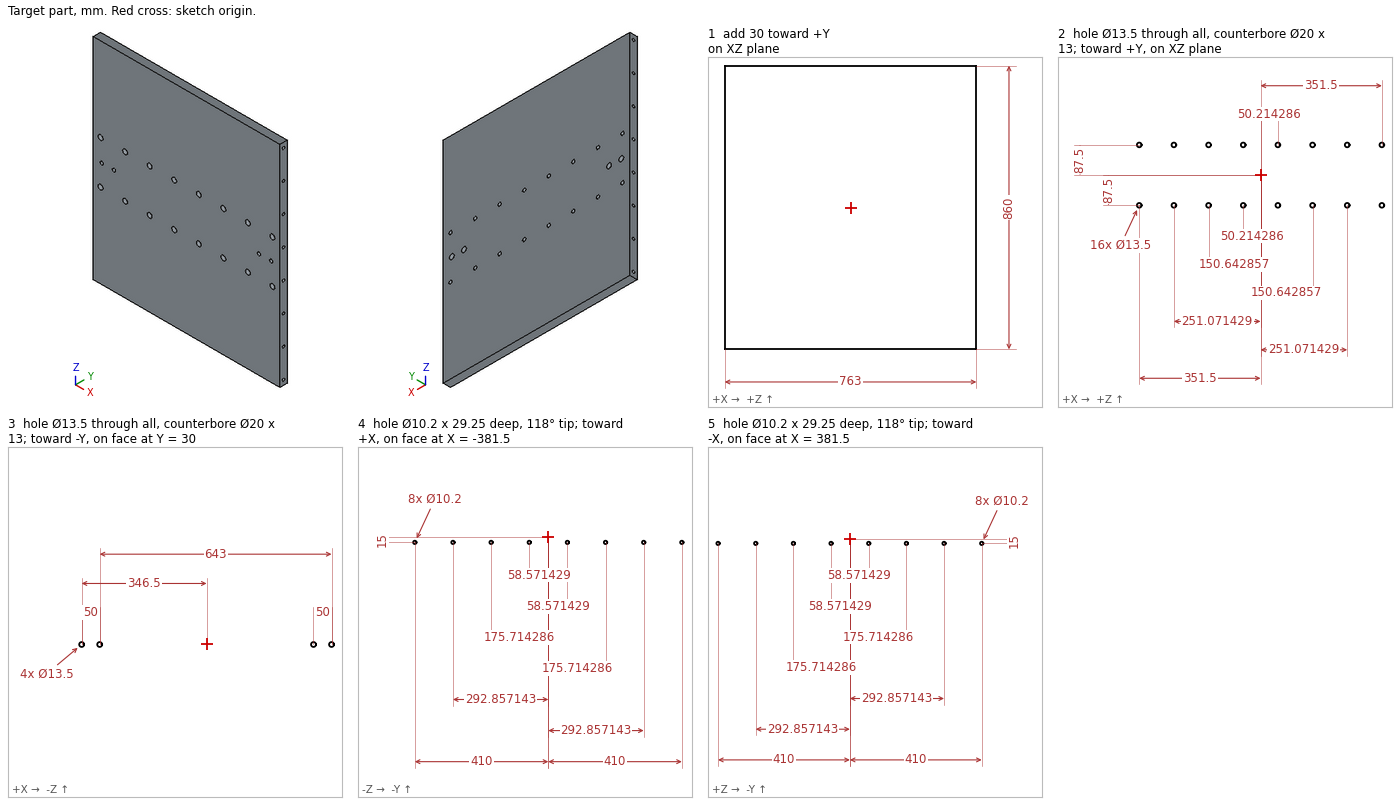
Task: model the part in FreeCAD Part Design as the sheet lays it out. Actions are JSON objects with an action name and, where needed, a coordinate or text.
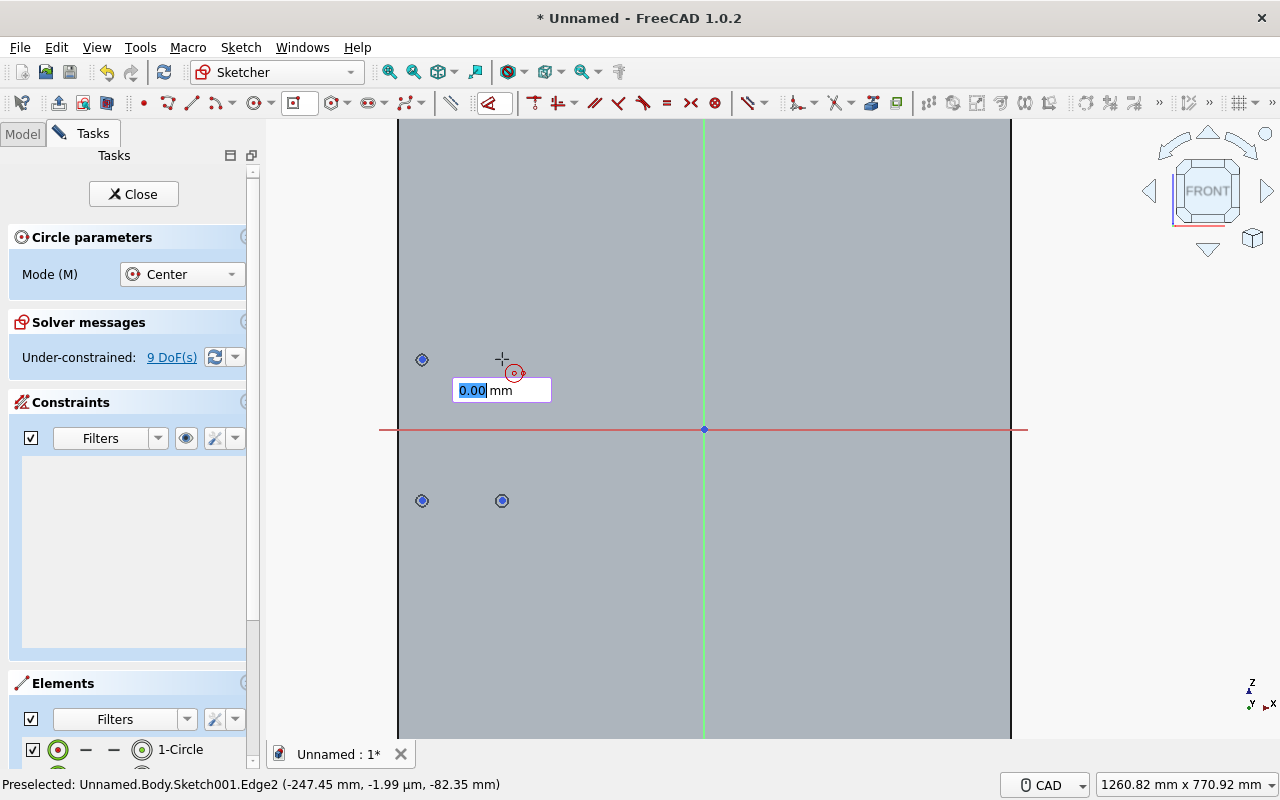
{"action": "scroll", "coordinate": [506, 355], "scroll_direction": "up", "scroll_amount": 6}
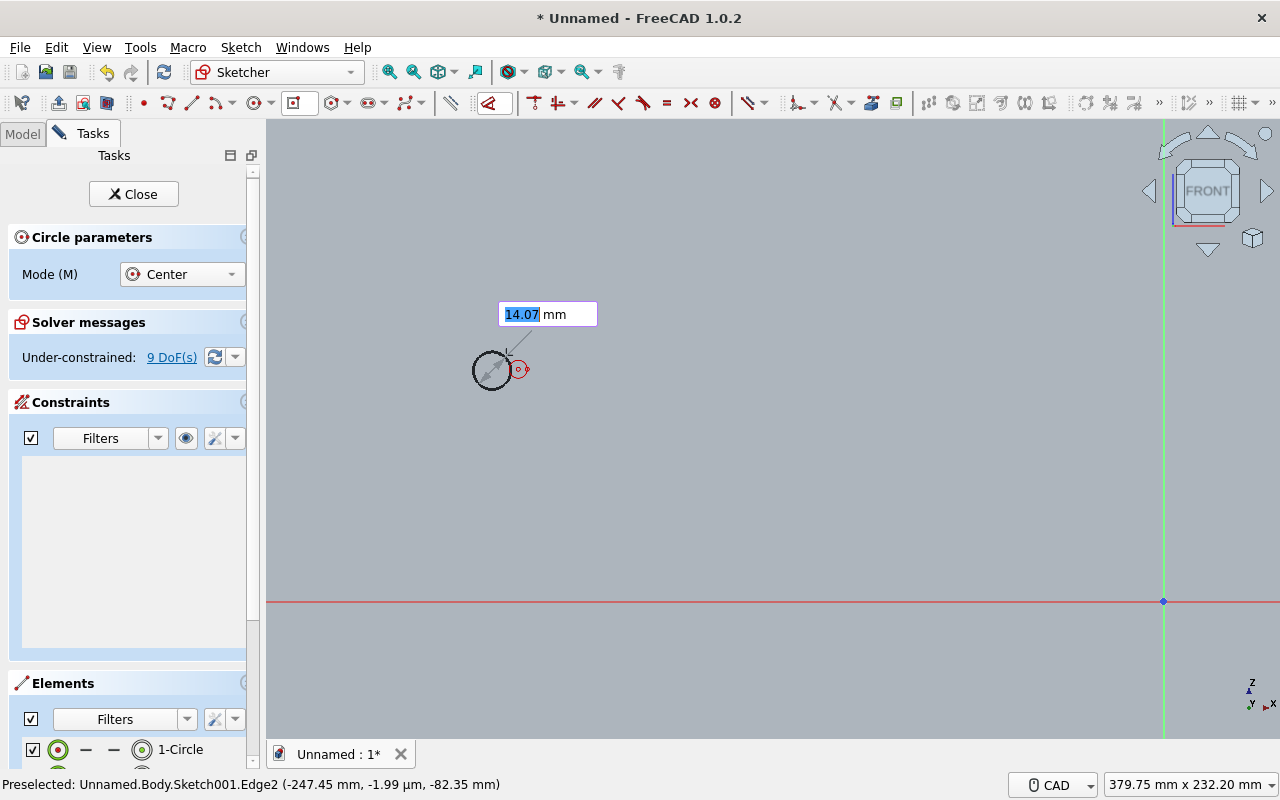
{"action": "left_click", "coordinate": [506, 355]}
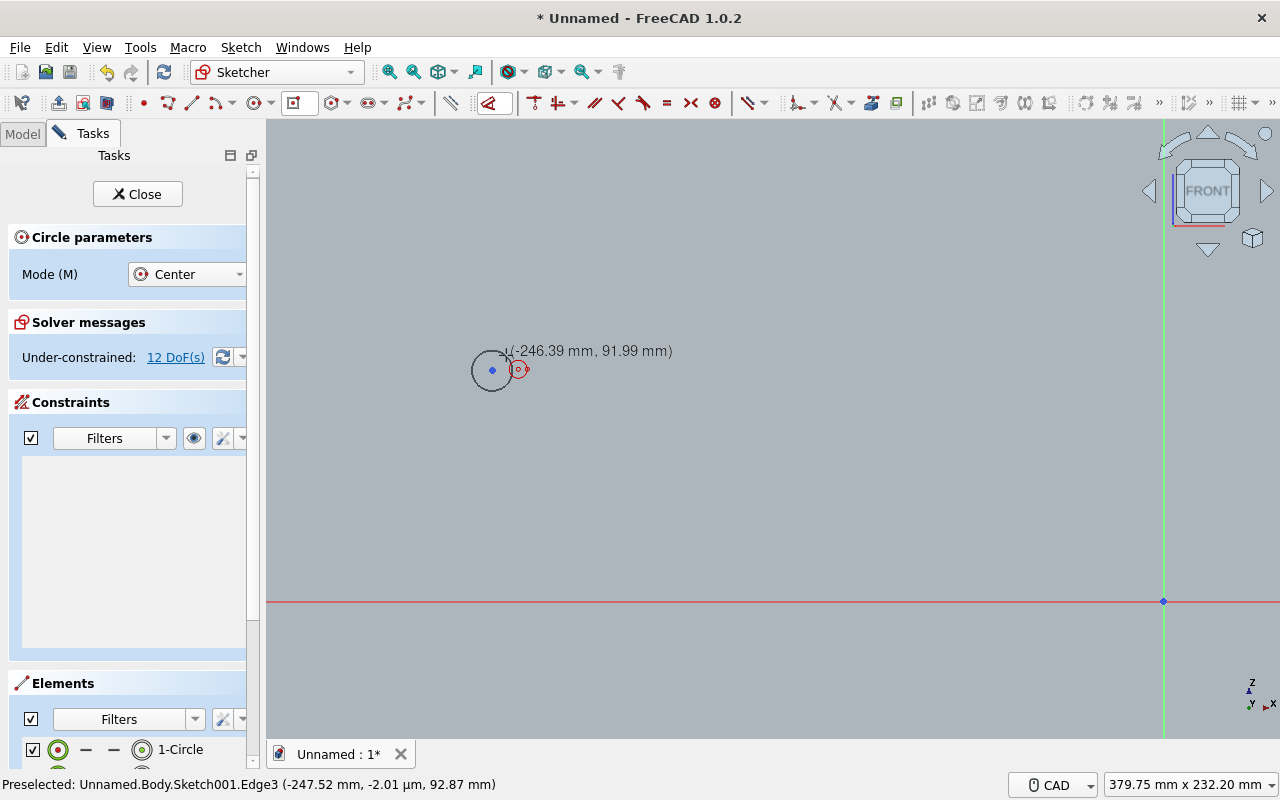
{"action": "scroll", "coordinate": [506, 355], "scroll_direction": "down", "scroll_amount": 6}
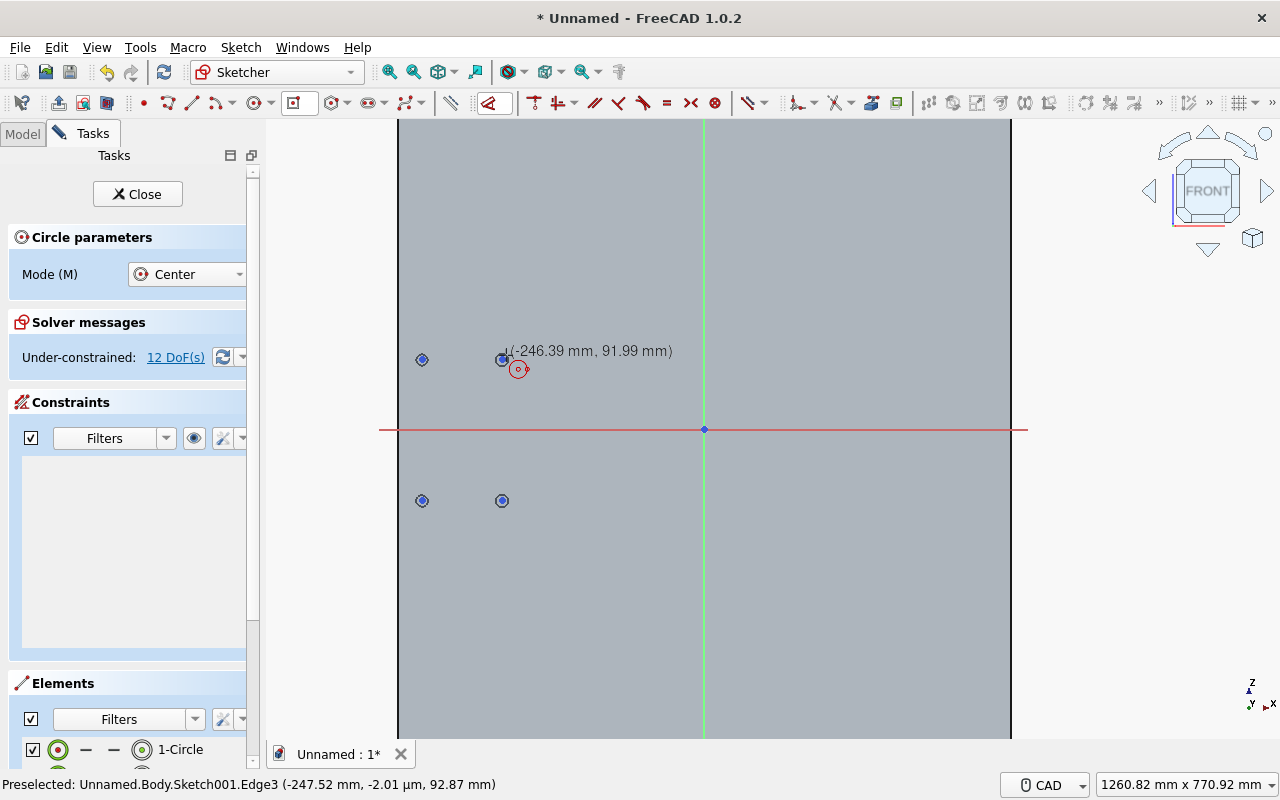
{"action": "scroll", "coordinate": [583, 500], "scroll_direction": "up", "scroll_amount": 8}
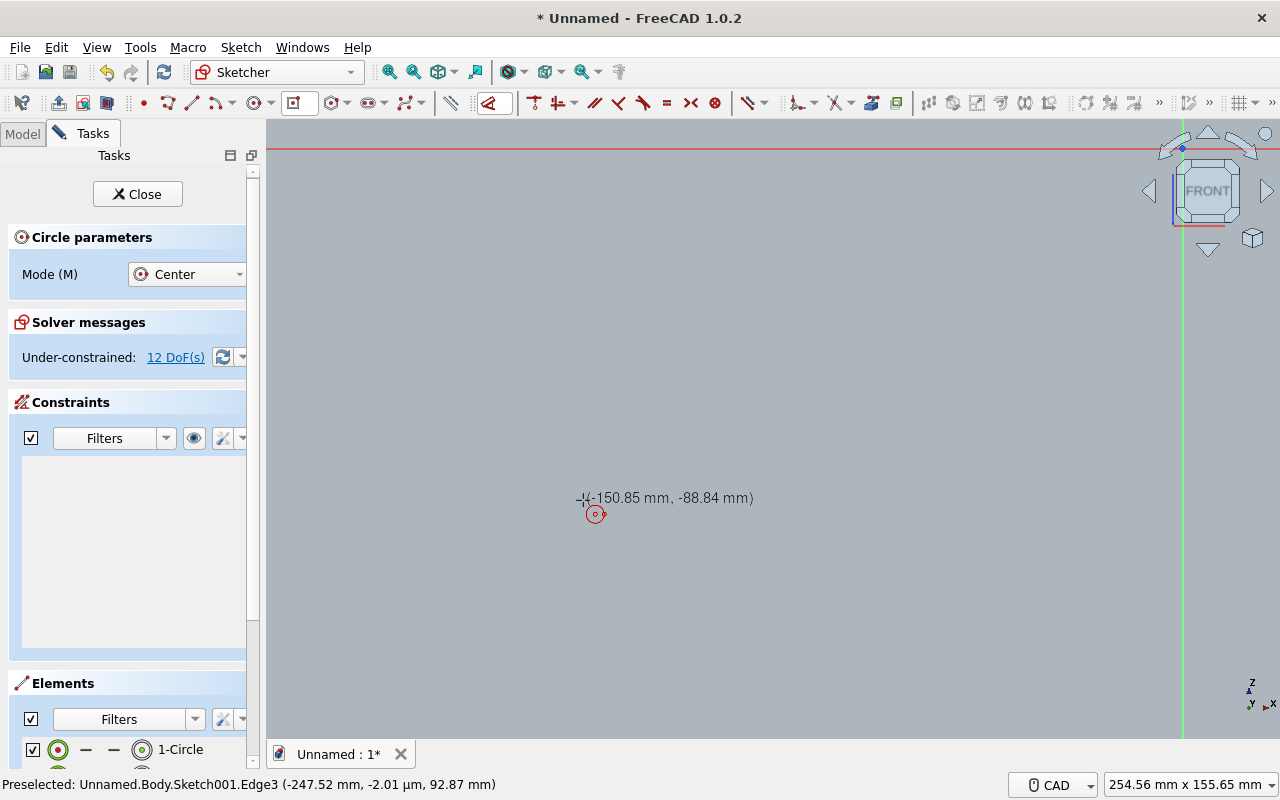
{"action": "scroll", "coordinate": [584, 500], "scroll_direction": "down", "scroll_amount": 8}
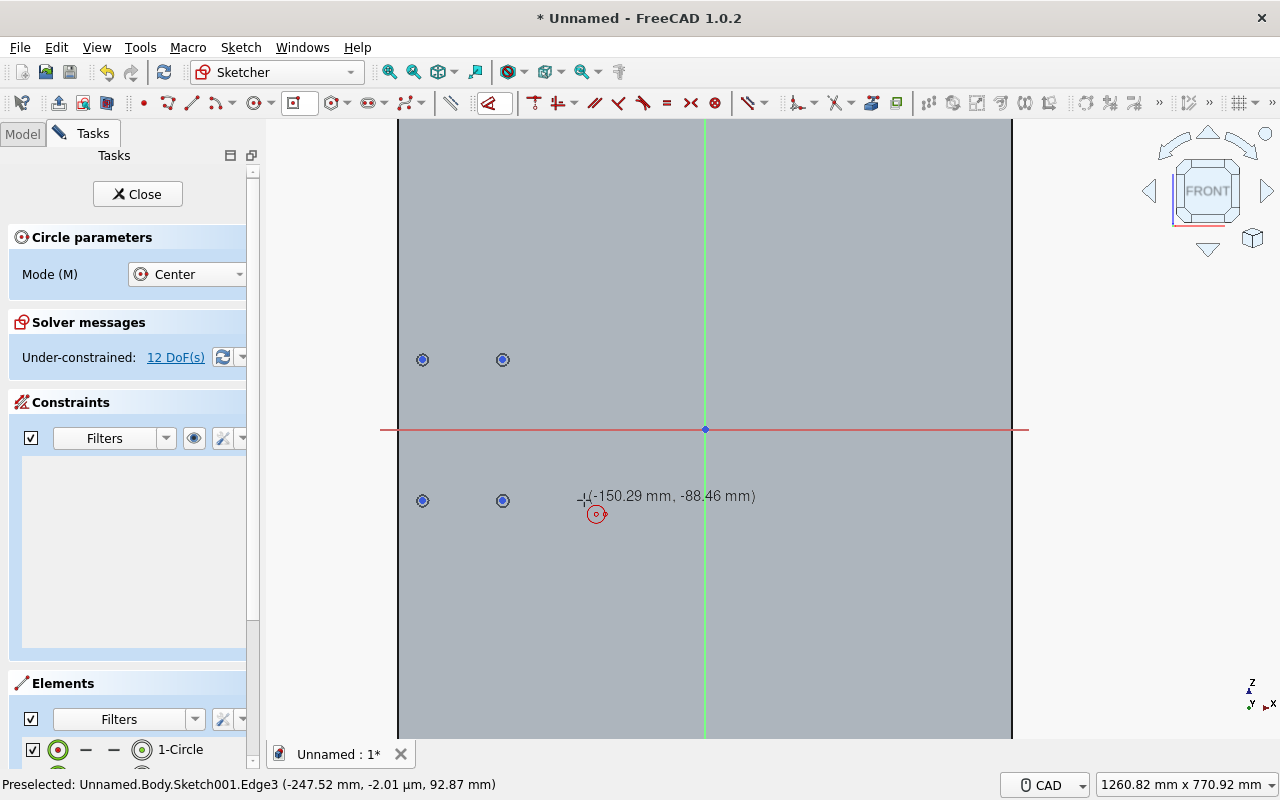
{"action": "left_click", "coordinate": [584, 500]}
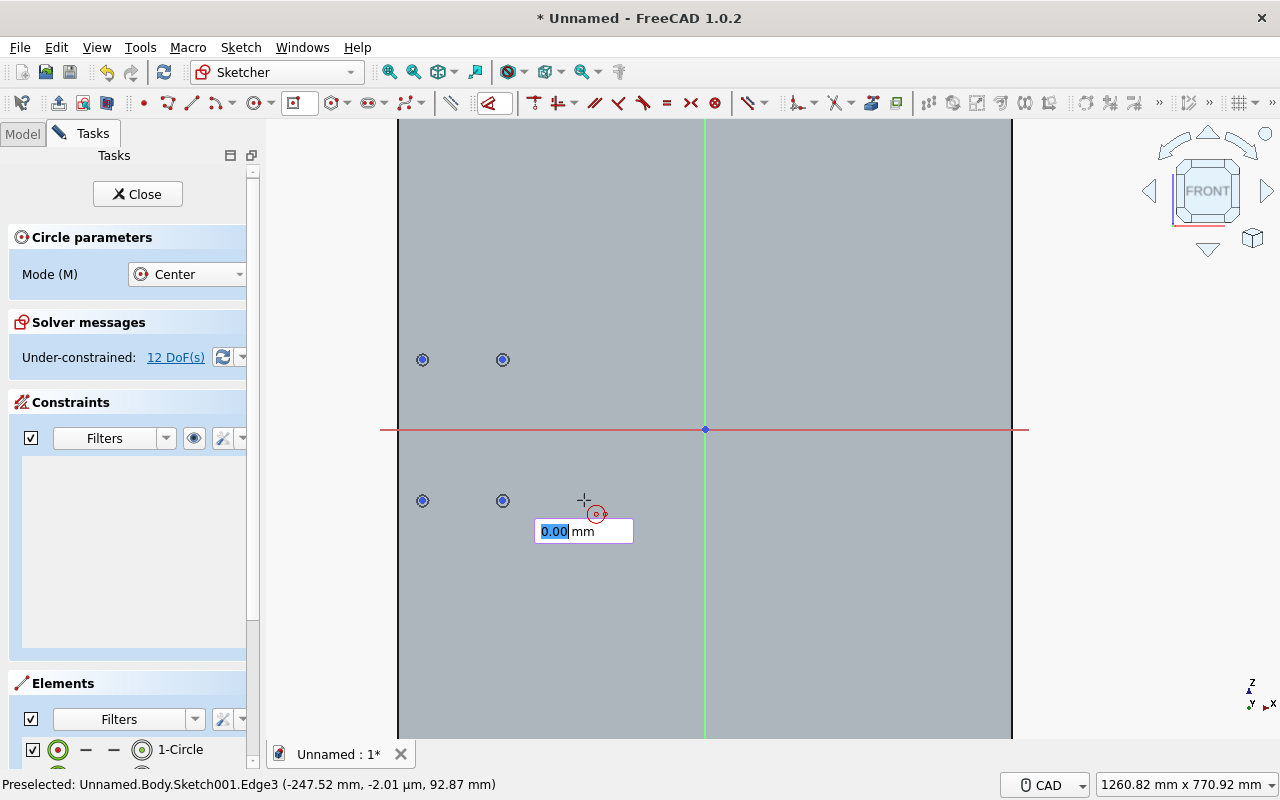
{"action": "scroll", "coordinate": [588, 496], "scroll_direction": "up", "scroll_amount": 6}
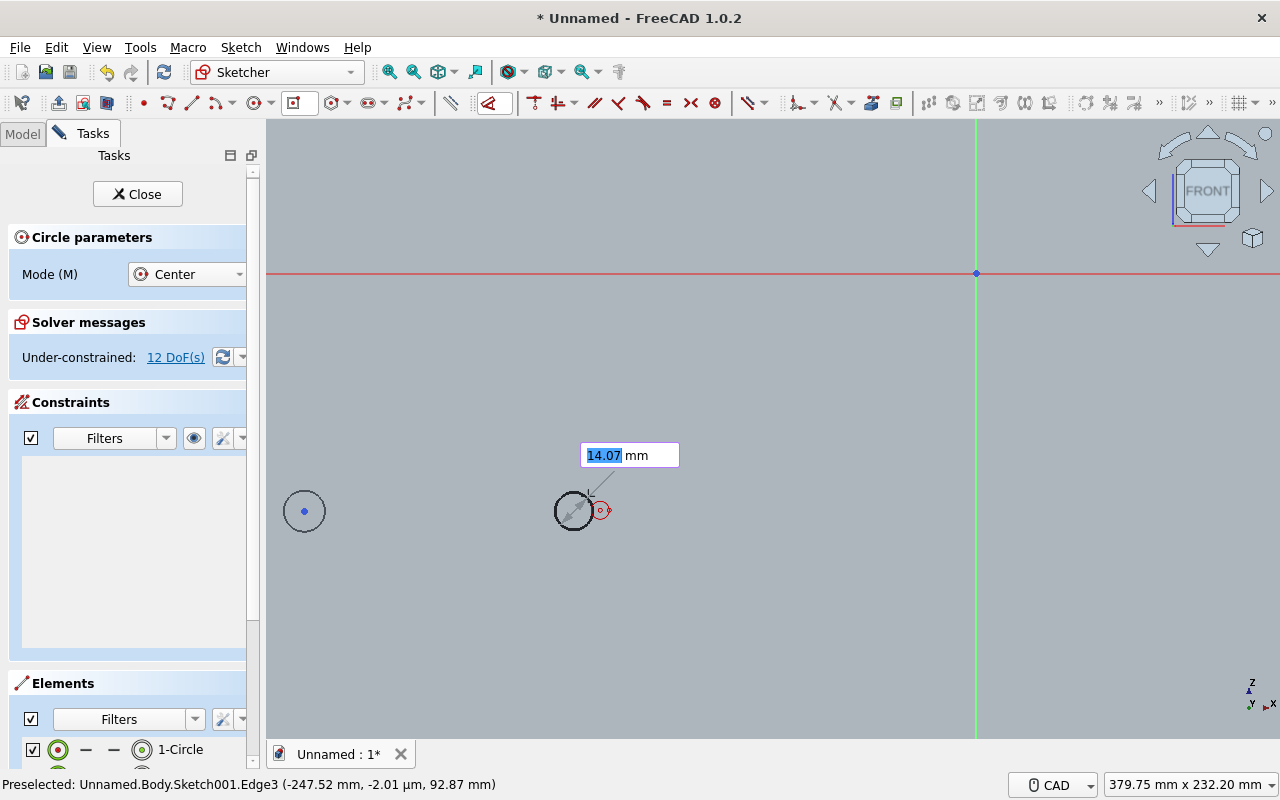
{"action": "left_click", "coordinate": [587, 495]}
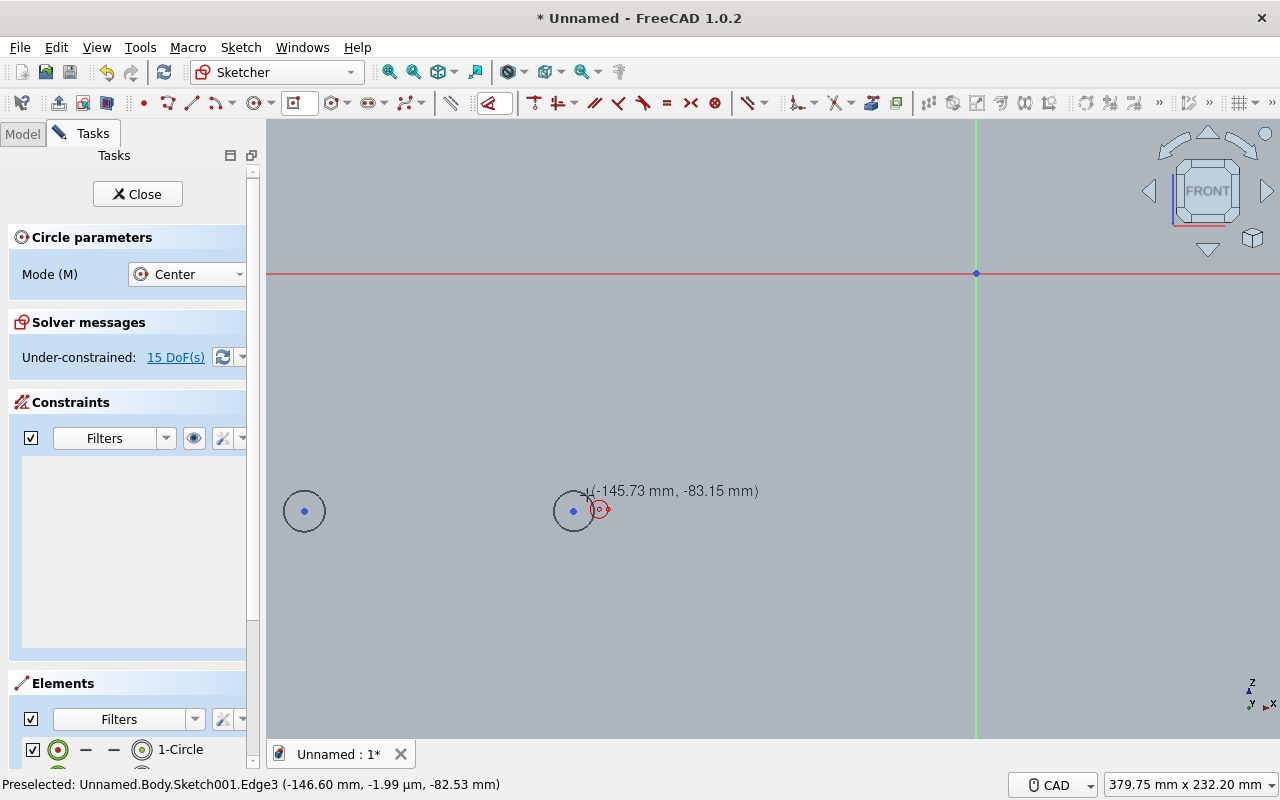
{"action": "scroll", "coordinate": [587, 496], "scroll_direction": "down", "scroll_amount": 6}